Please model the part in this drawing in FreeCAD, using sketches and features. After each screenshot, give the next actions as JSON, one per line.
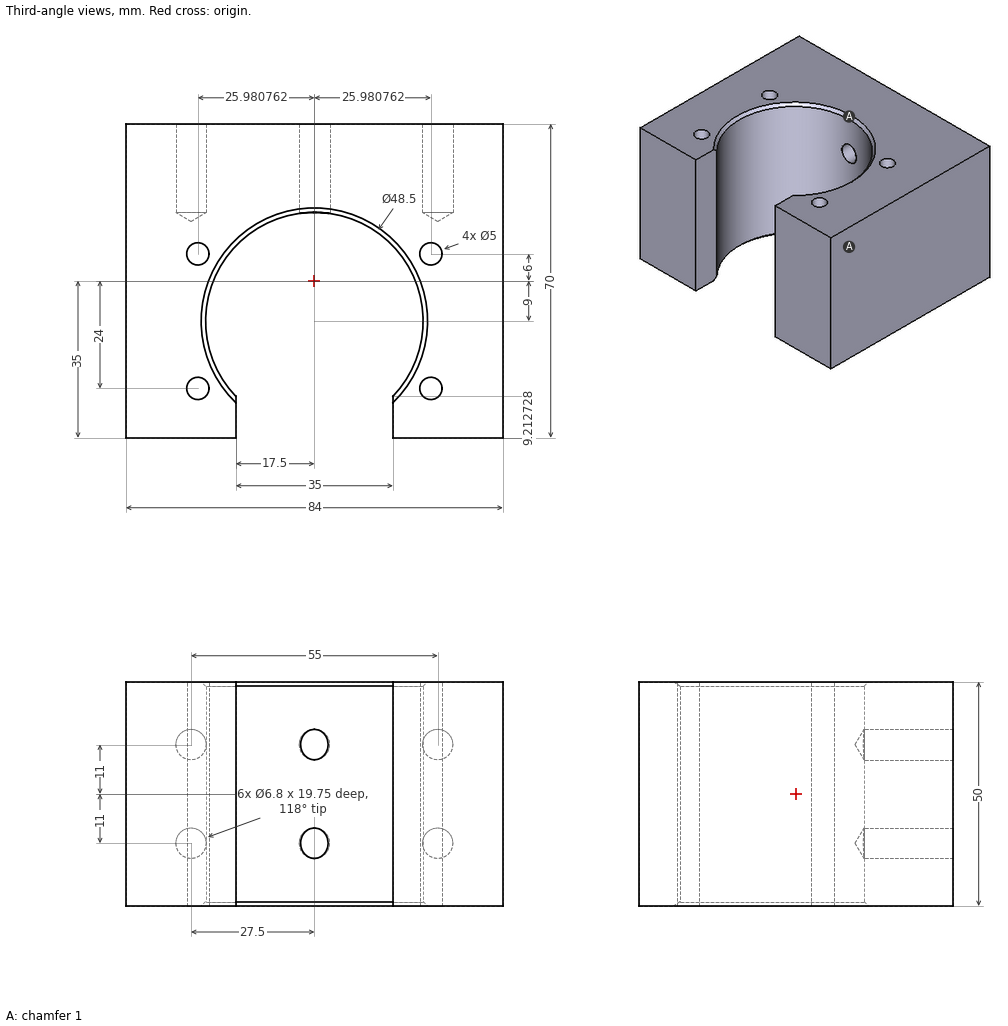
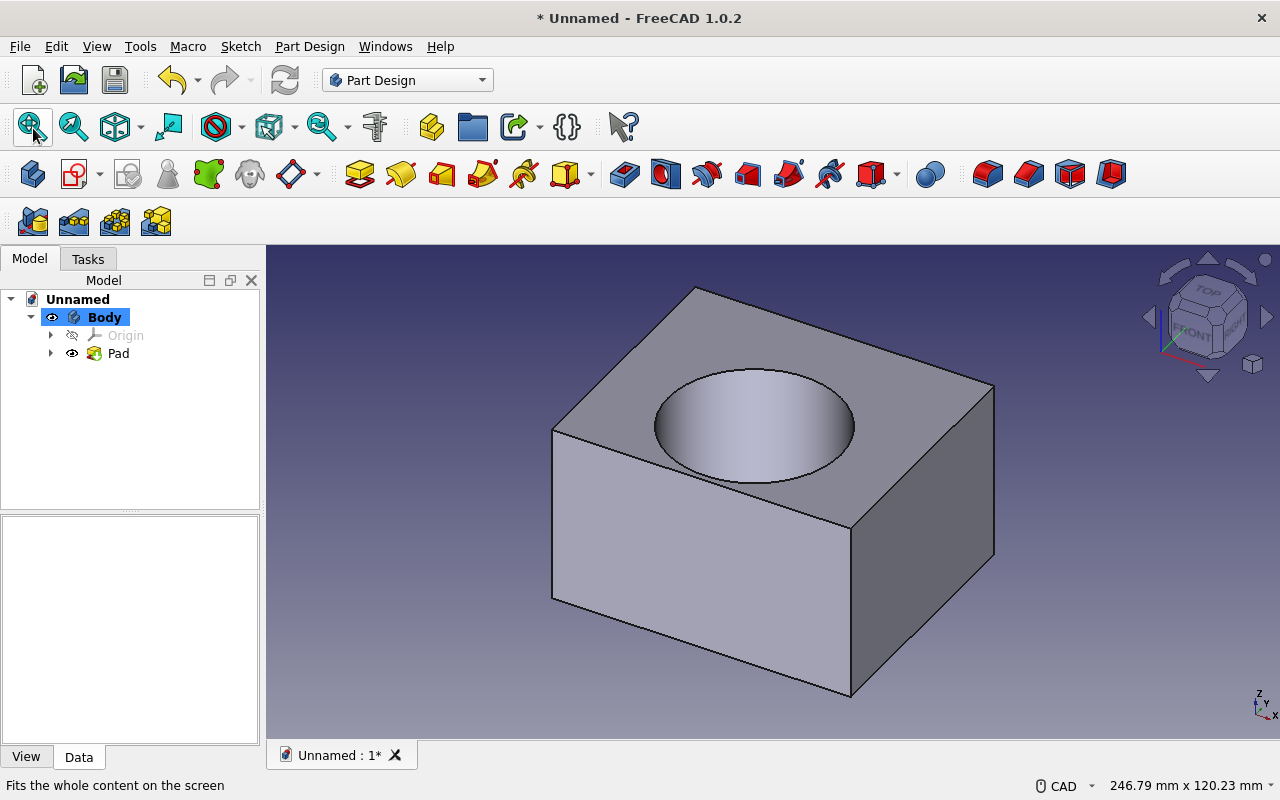
{"action": "left_click", "coordinate": [899, 394]}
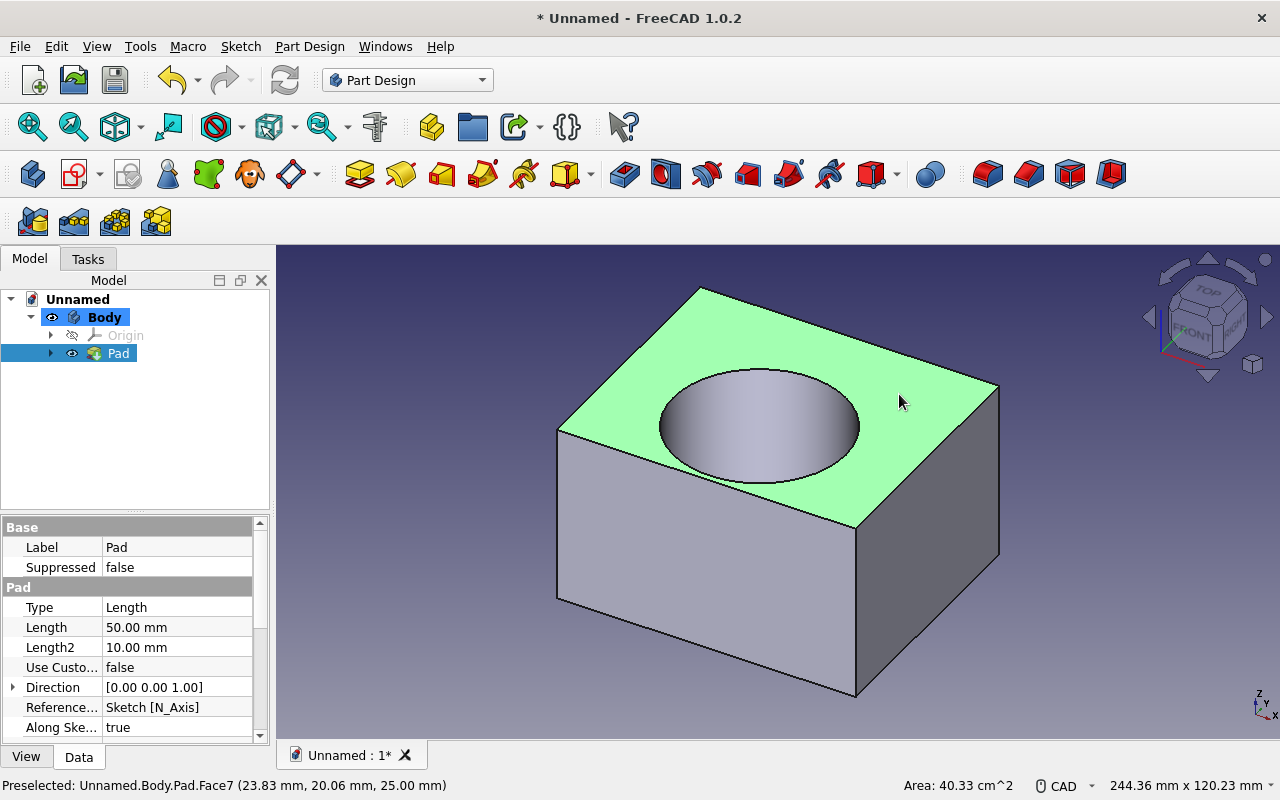
{"action": "left_click", "coordinate": [74, 174]}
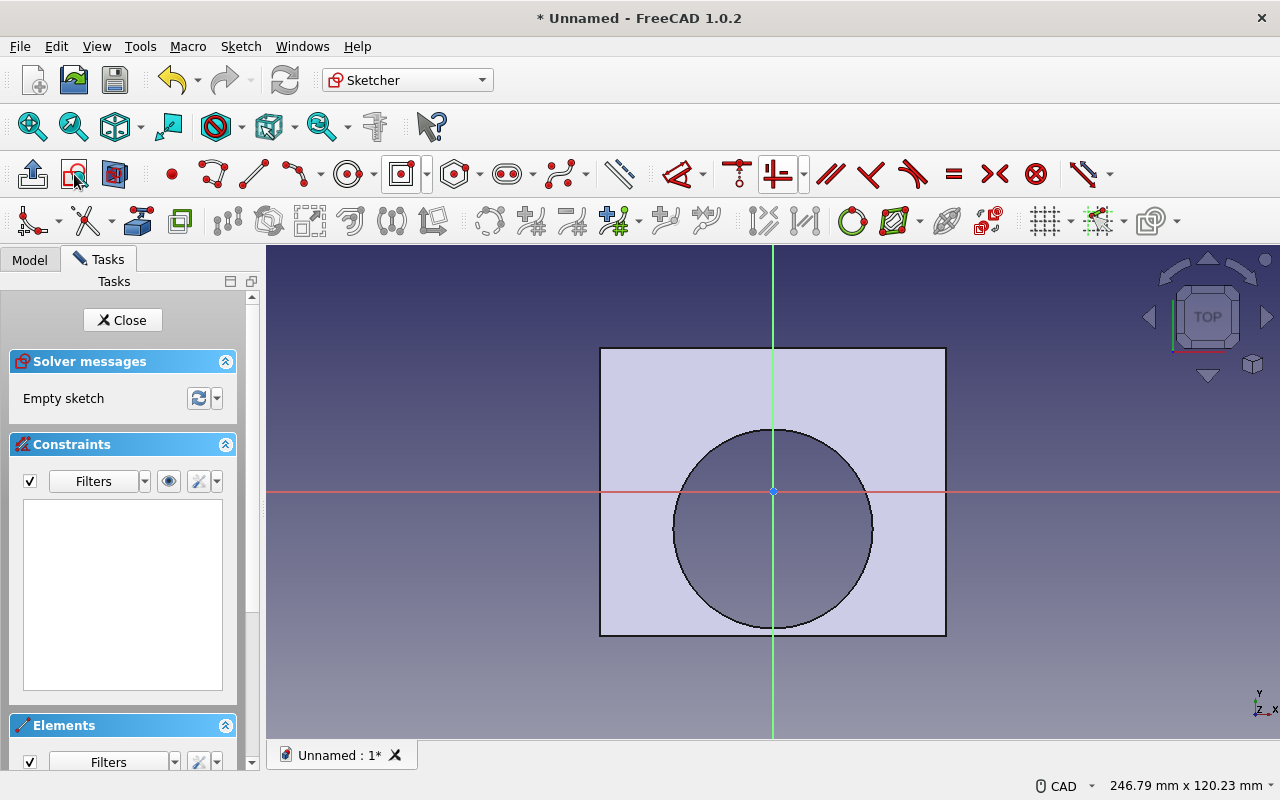
{"action": "scroll", "coordinate": [829, 623], "scroll_direction": "up", "scroll_amount": 4}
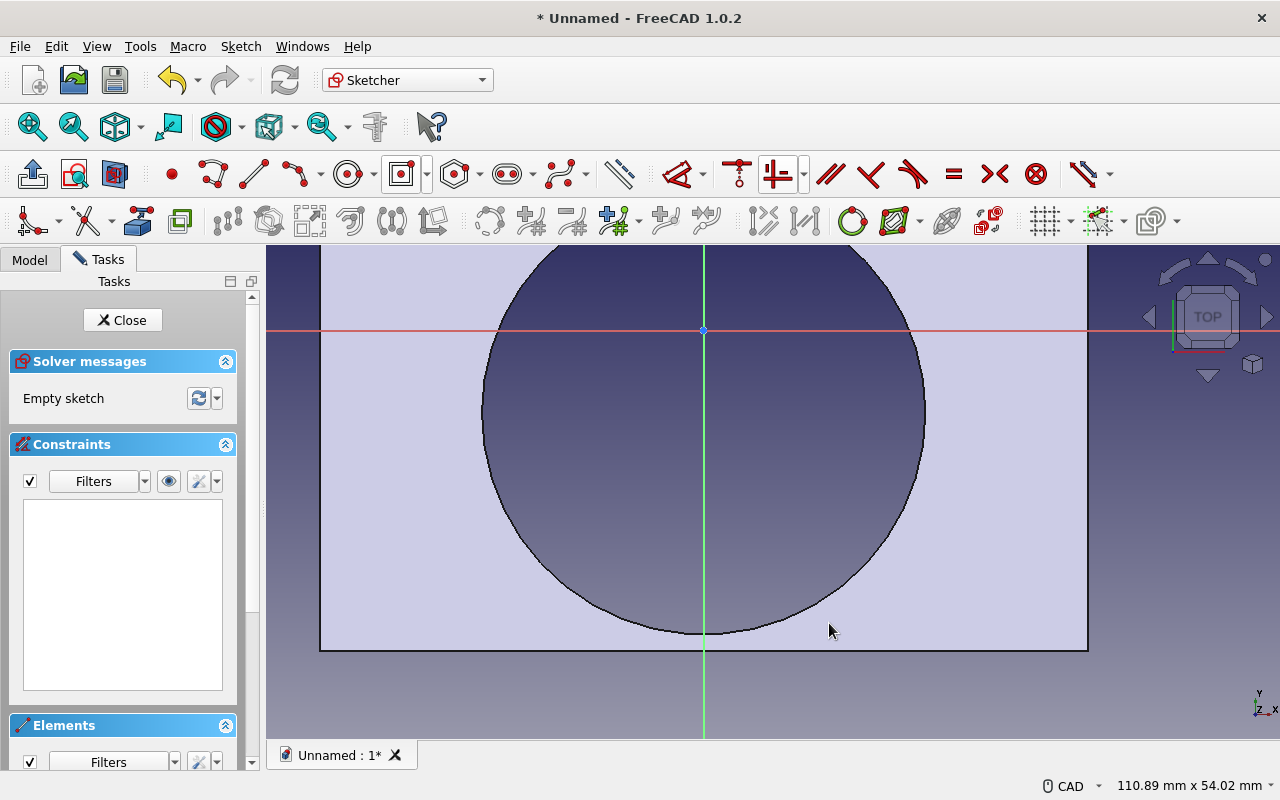
{"action": "left_click", "coordinate": [426, 174]}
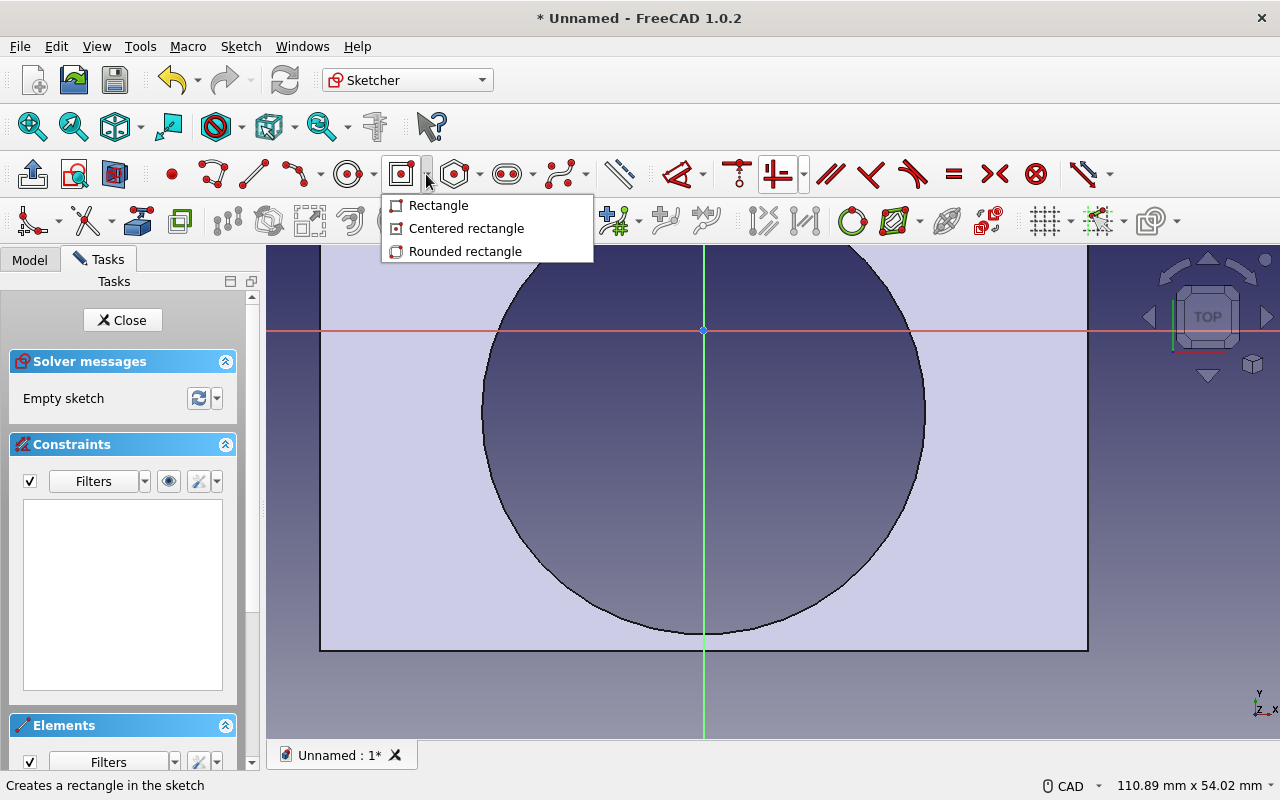
{"action": "left_click", "coordinate": [488, 206]}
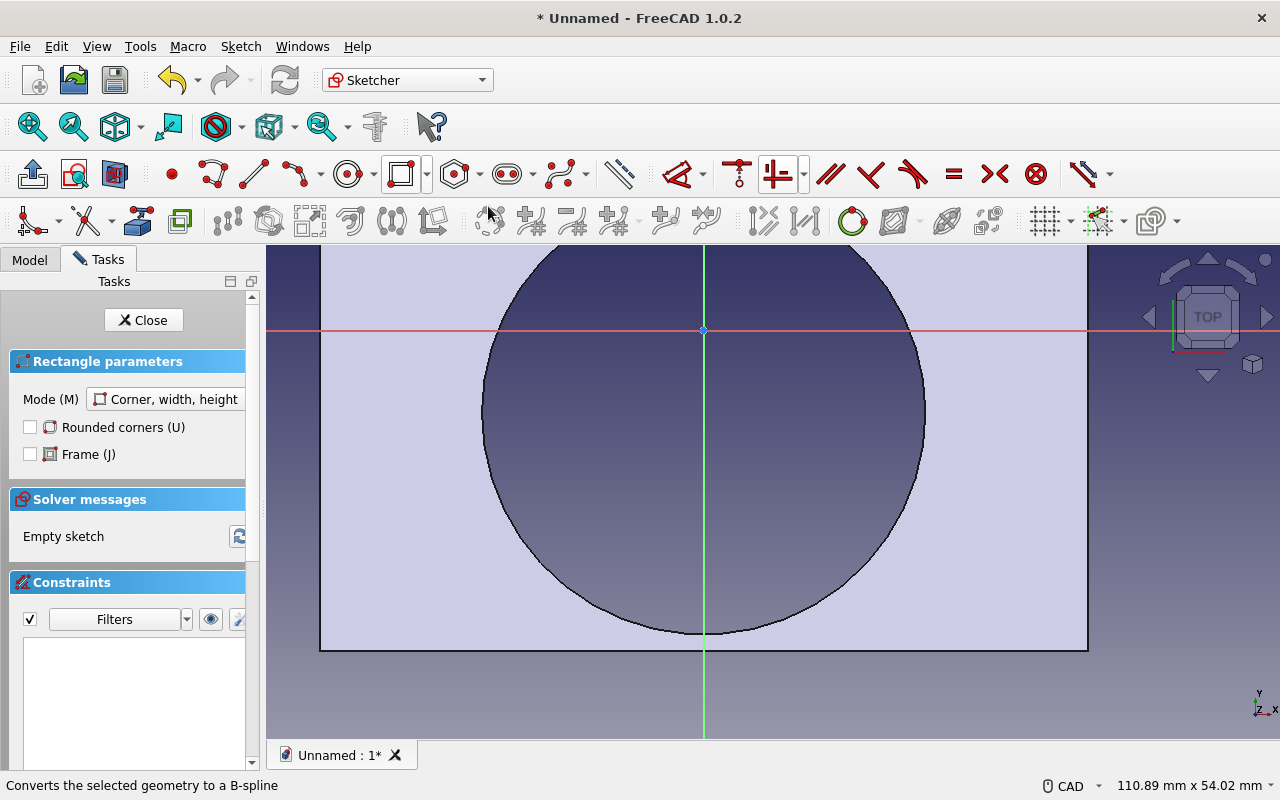
{"action": "left_click", "coordinate": [544, 566]}
{"action": "mouse_move", "coordinate": [864, 651]}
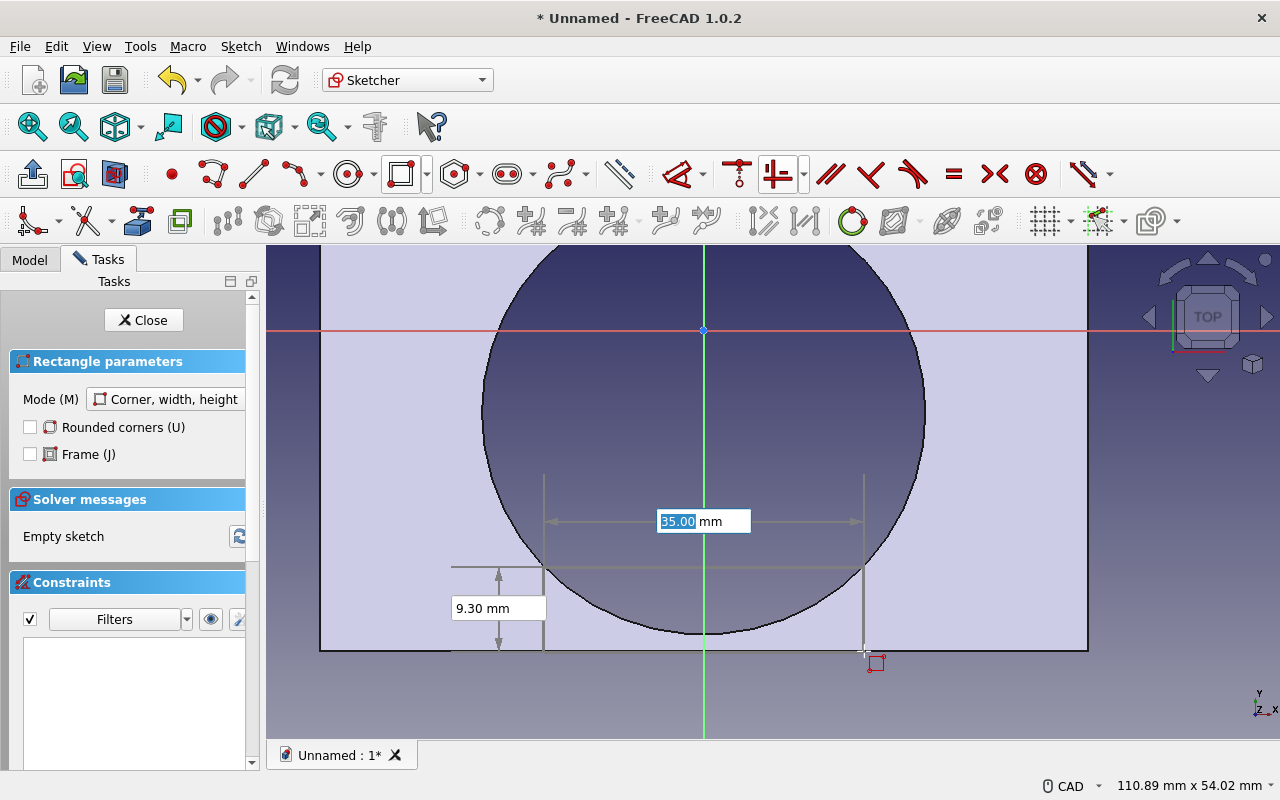
{"action": "type", "text": "35"}
{"action": "key", "text": "Tab"}
{"action": "type", "text": "9.212728"}
{"action": "key", "text": "Return"}
{"action": "key", "text": "Escape"}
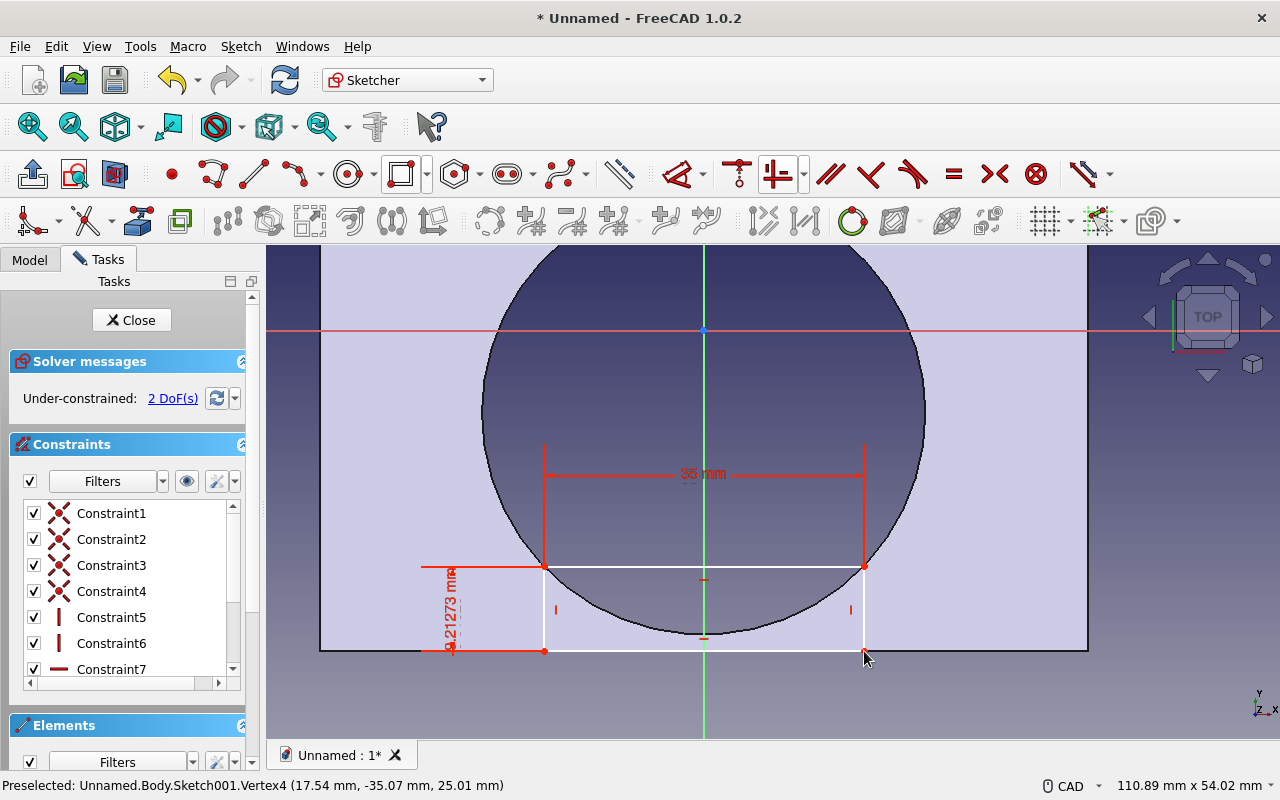
{"action": "left_click", "coordinate": [676, 174]}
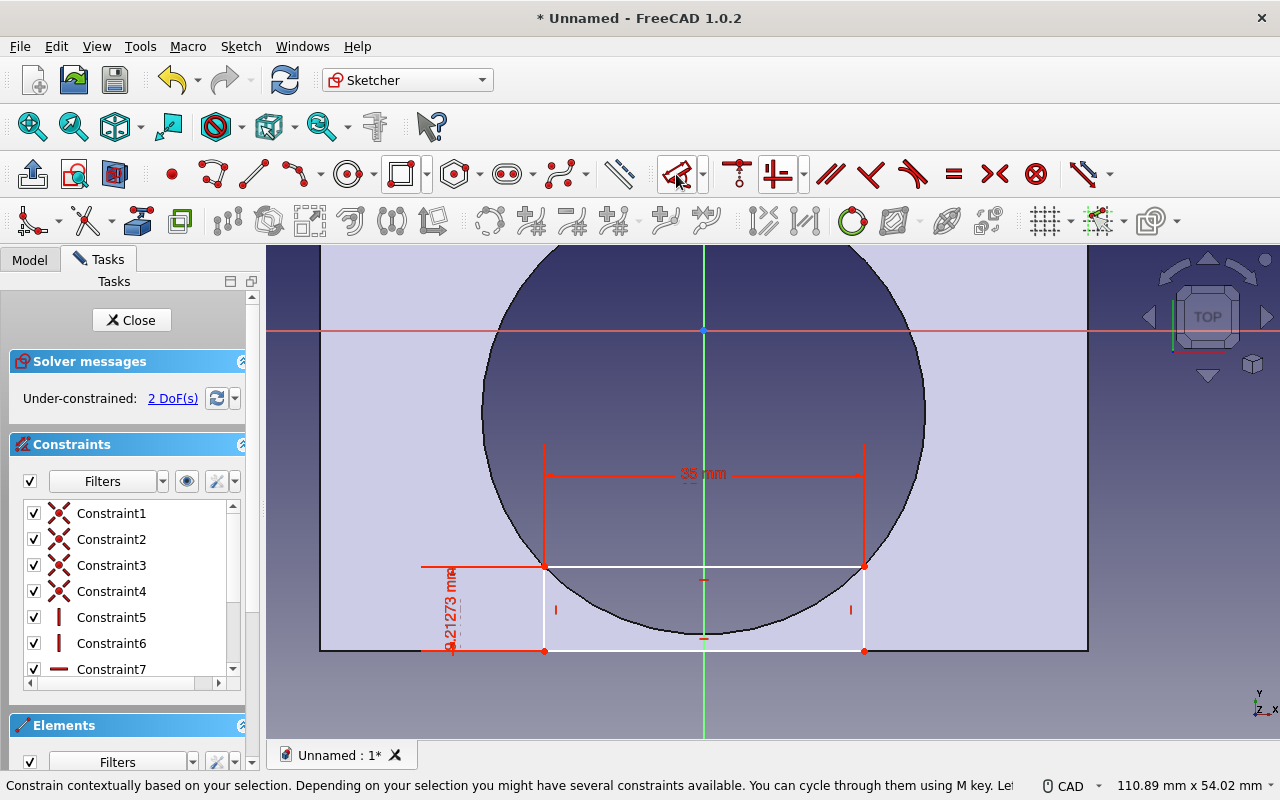
{"action": "left_click", "coordinate": [544, 651]}
{"action": "left_click", "coordinate": [510, 491]}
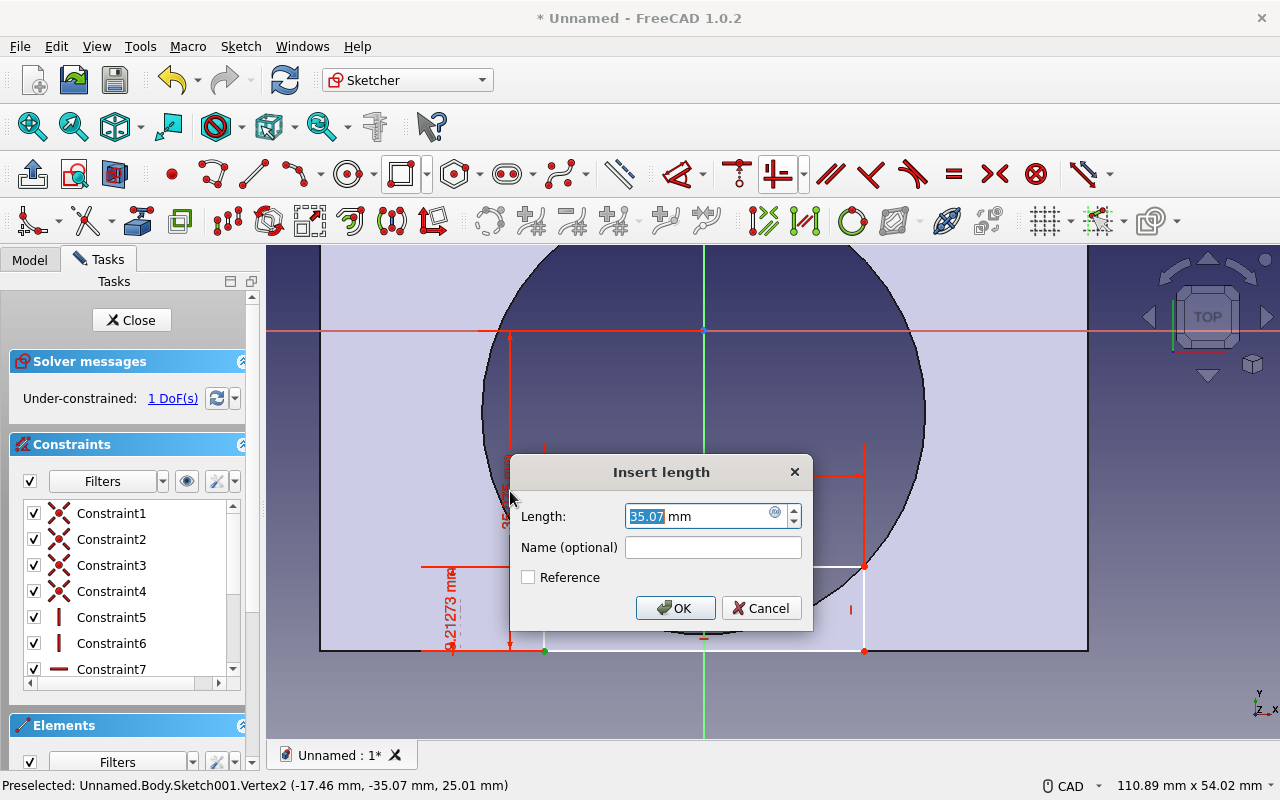
{"action": "type", "text": "35"}
{"action": "key", "text": "Return"}